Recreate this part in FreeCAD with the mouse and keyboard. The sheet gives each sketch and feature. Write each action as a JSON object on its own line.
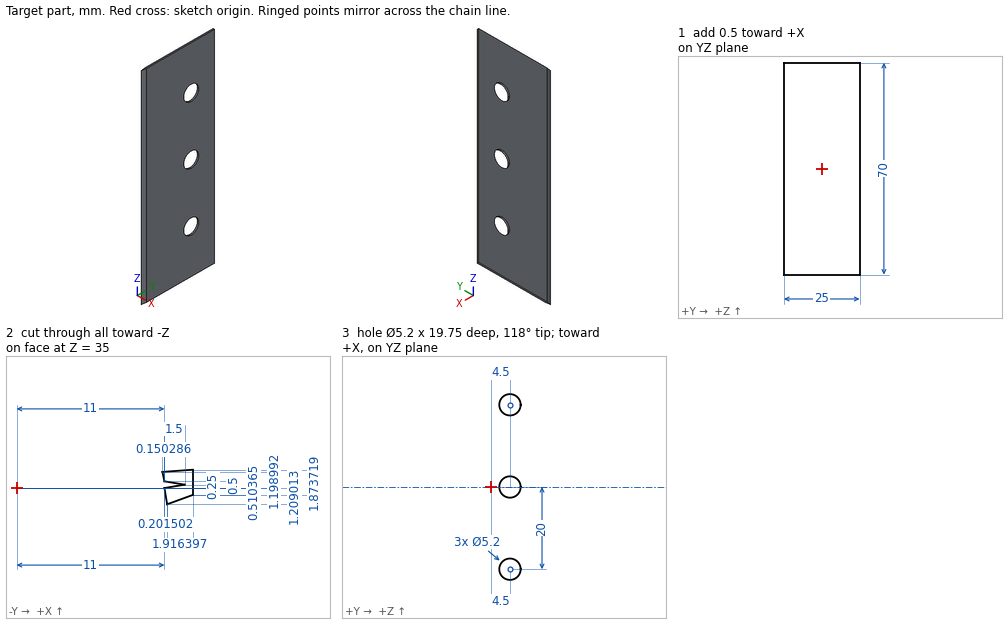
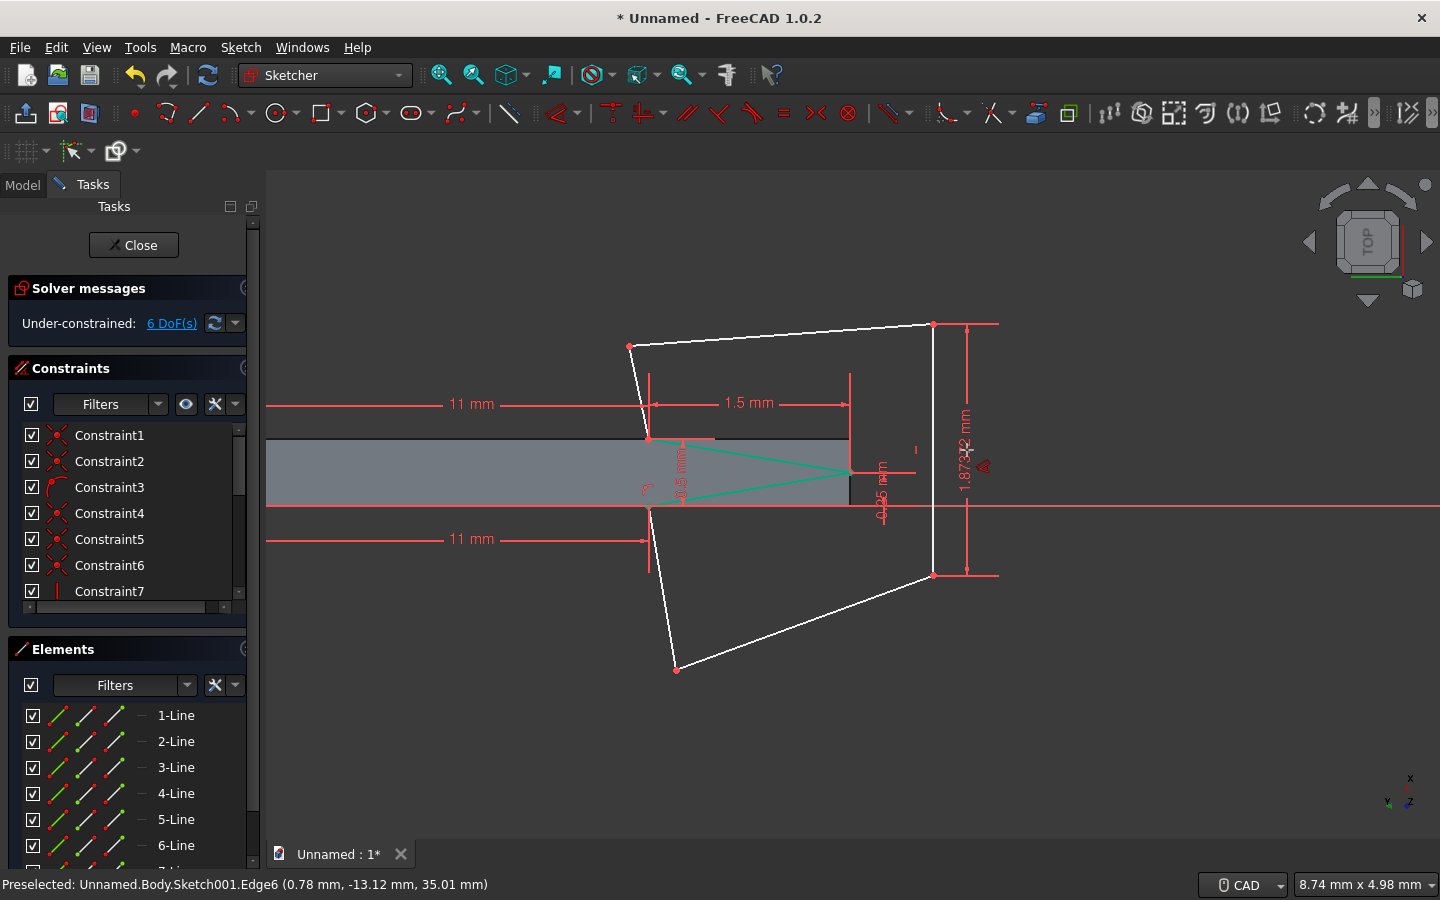
{"action": "left_click", "coordinate": [629, 346]}
{"action": "left_click", "coordinate": [663, 426]}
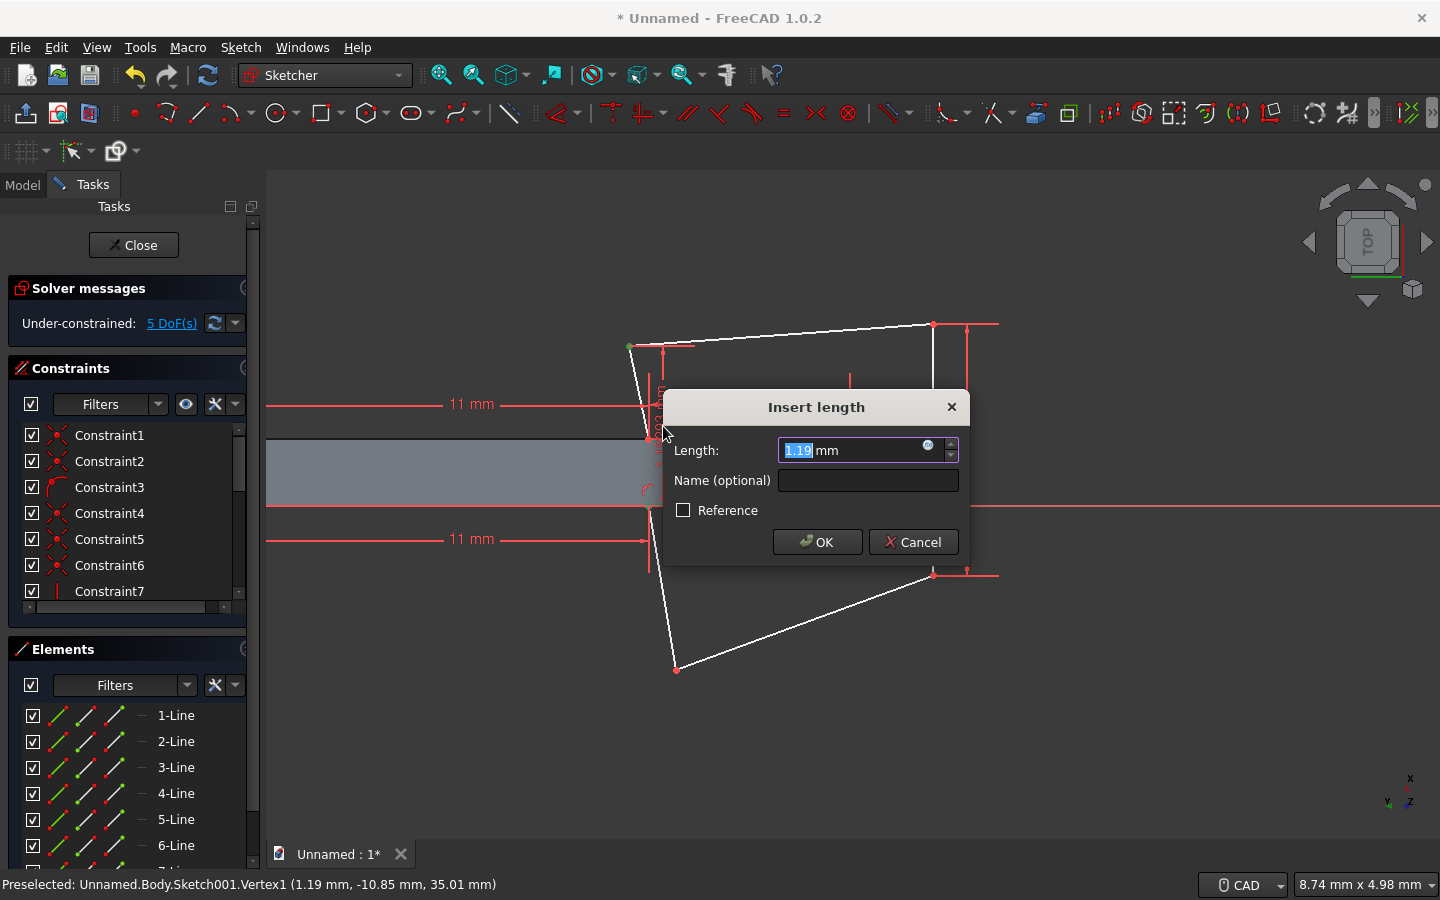
{"action": "type", "text": "1.198992"}
{"action": "key", "text": "Return"}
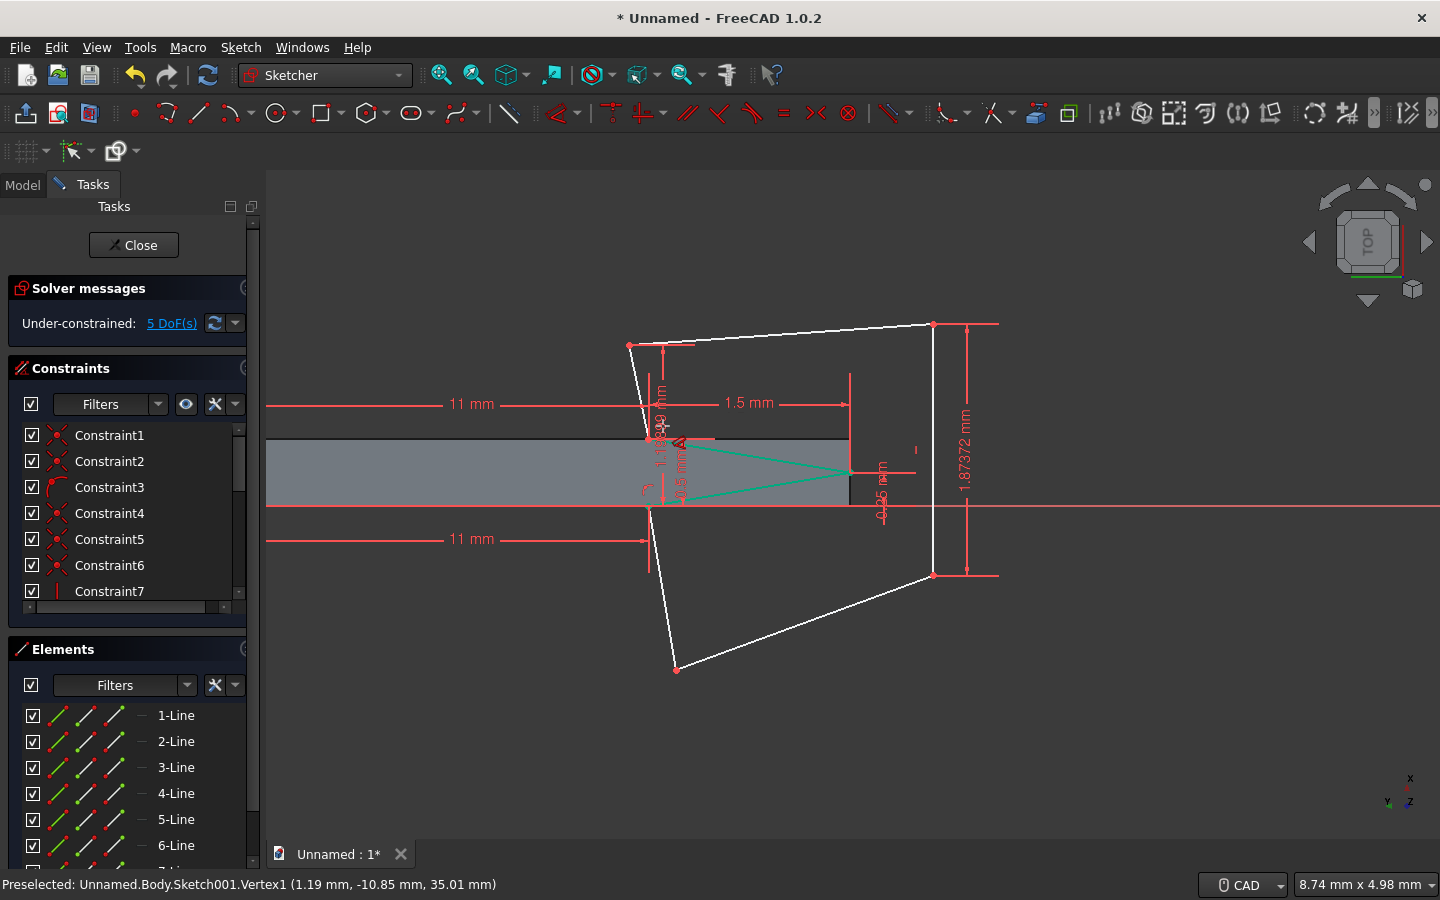
{"action": "left_click", "coordinate": [676, 670]}
{"action": "left_click", "coordinate": [710, 588]}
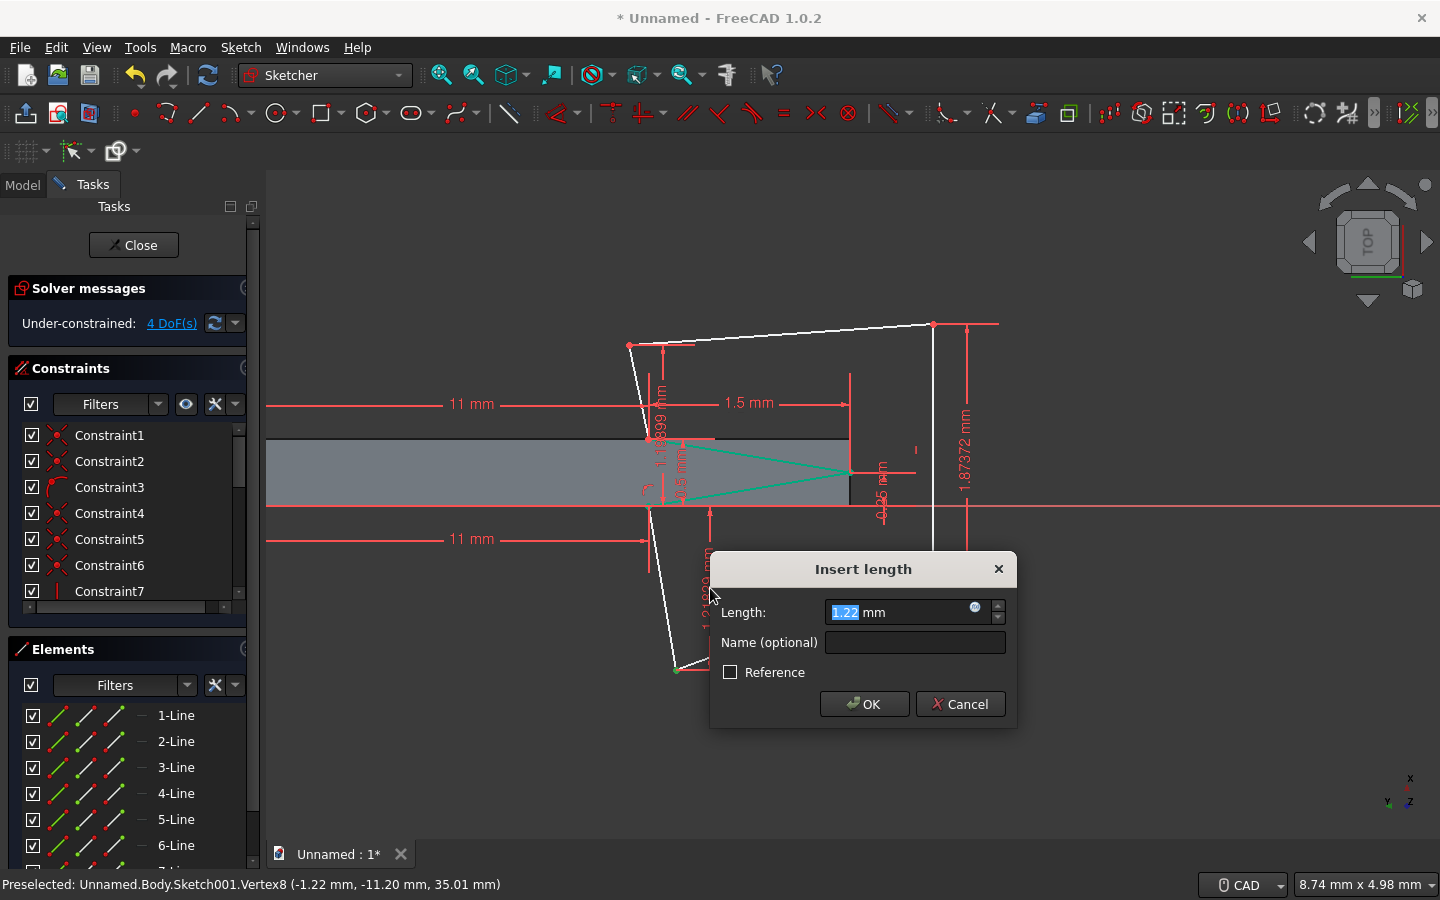
{"action": "type", "text": "1.209013"}
{"action": "key", "text": "Return"}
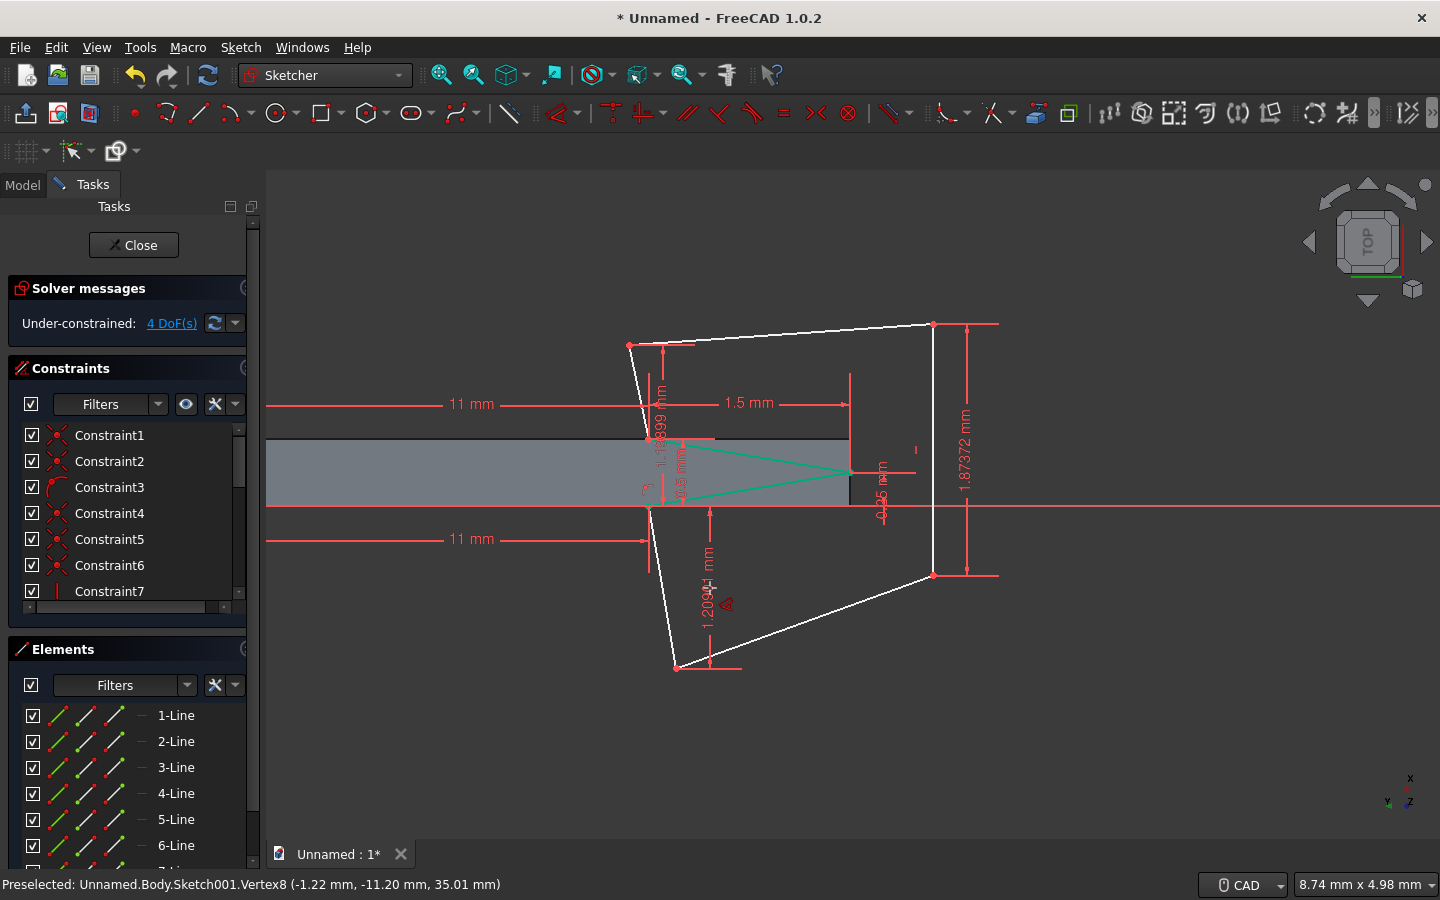
{"action": "left_click", "coordinate": [933, 576]}
{"action": "left_click", "coordinate": [967, 541]}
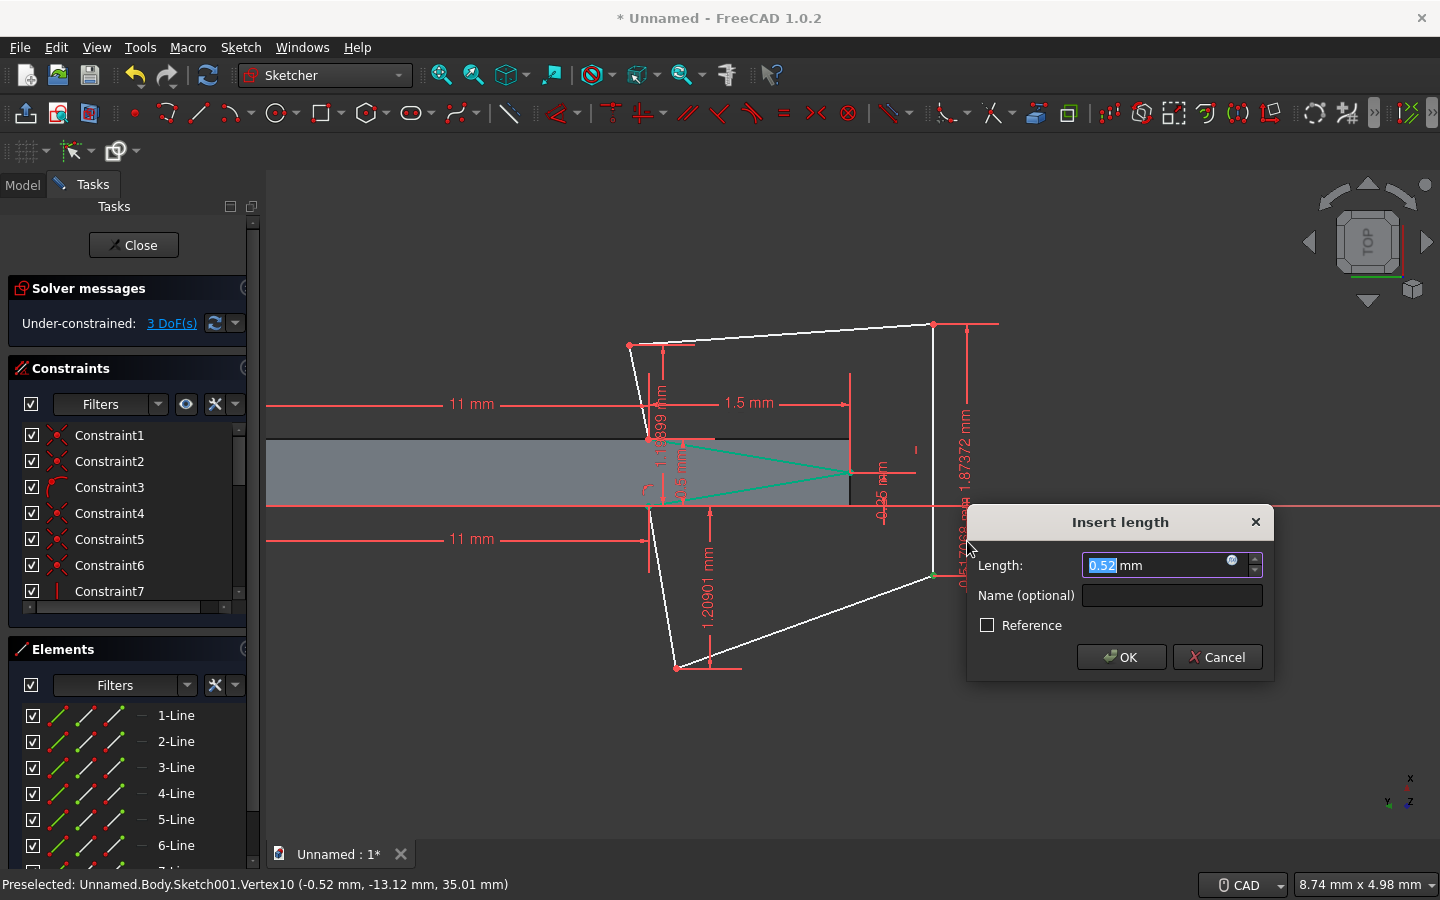
{"action": "type", "text": "0.510365"}
{"action": "key", "text": "Return"}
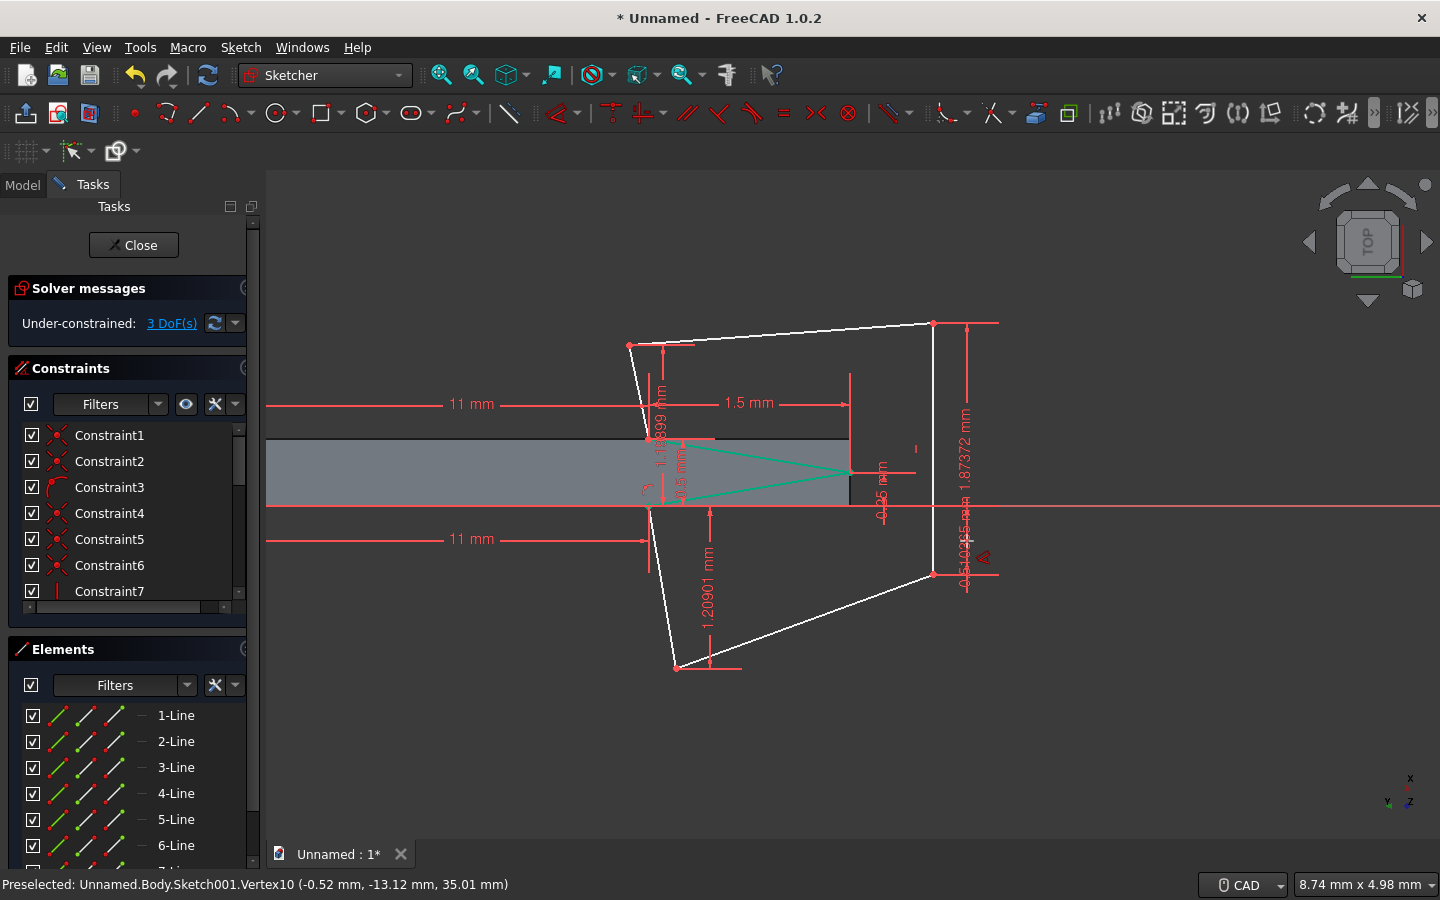
{"action": "scroll", "coordinate": [635, 373], "scroll_direction": "up", "scroll_amount": 4}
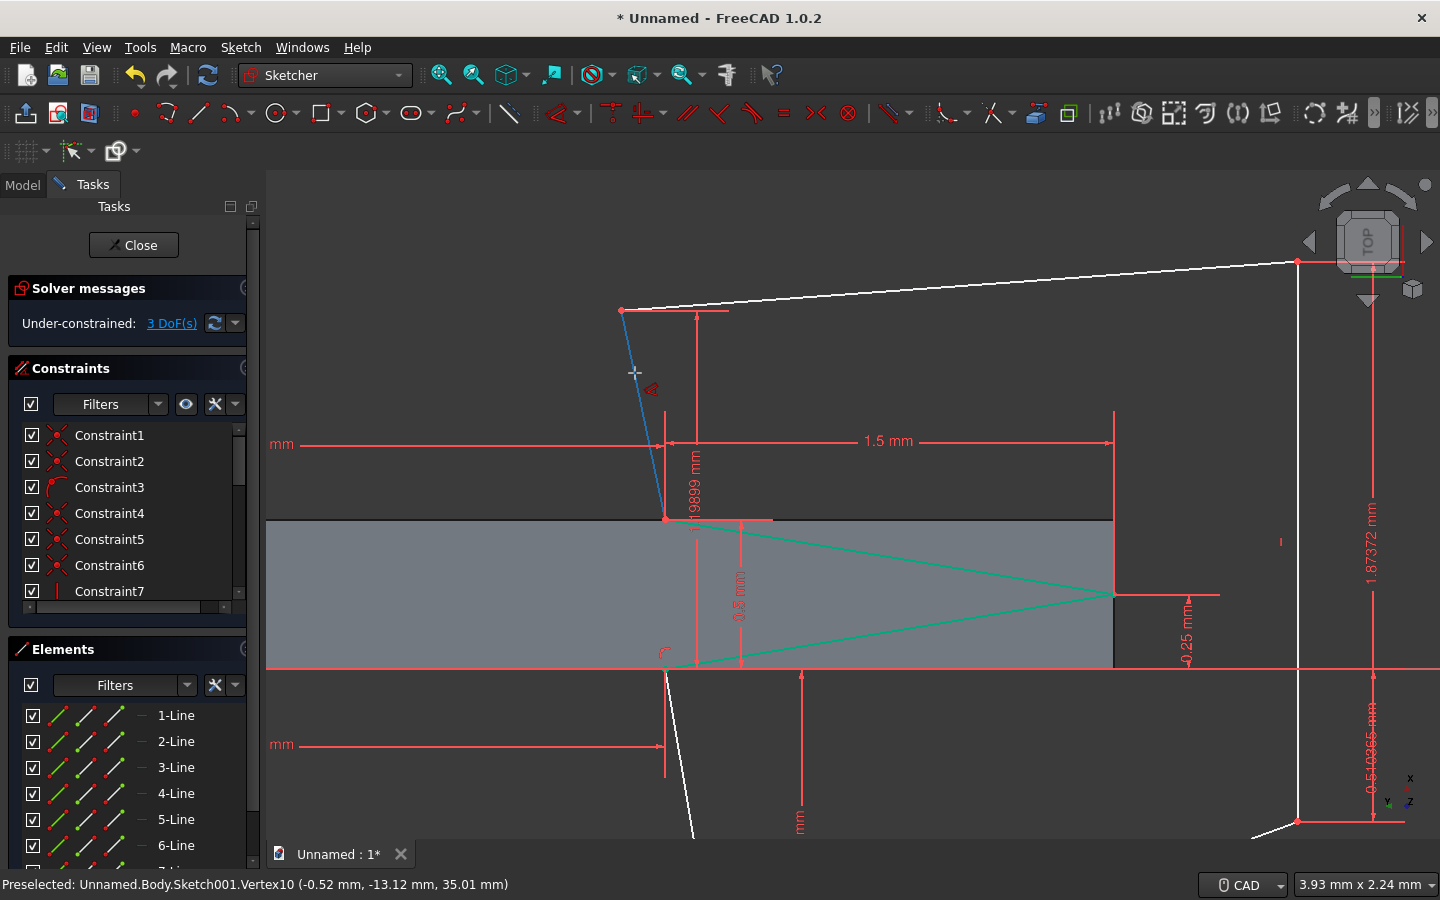
{"action": "left_click", "coordinate": [634, 373]}
{"action": "left_click", "coordinate": [643, 277]}